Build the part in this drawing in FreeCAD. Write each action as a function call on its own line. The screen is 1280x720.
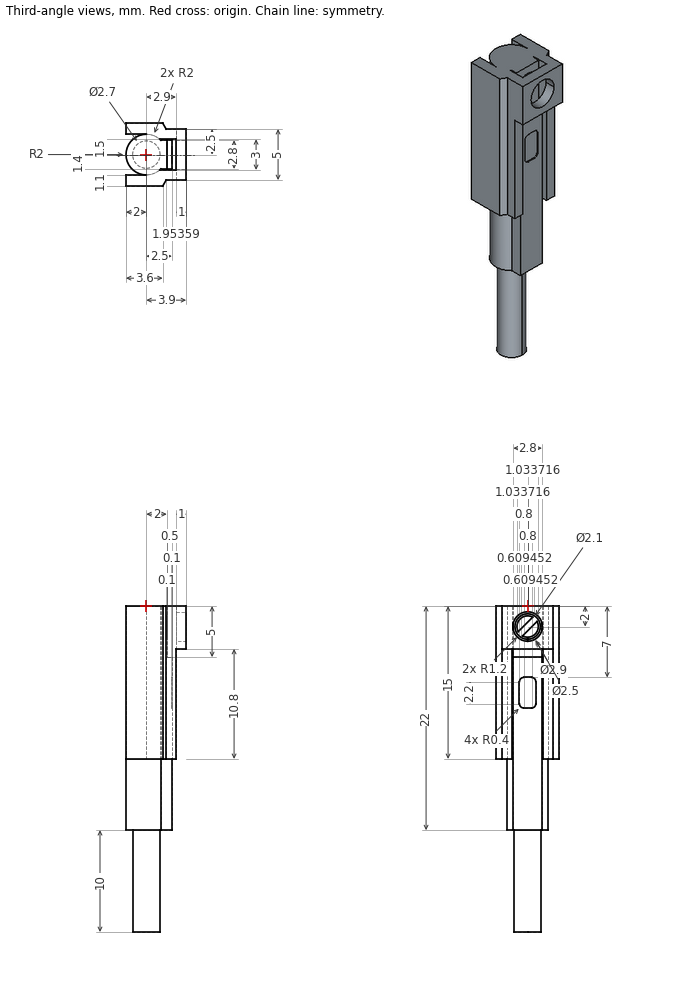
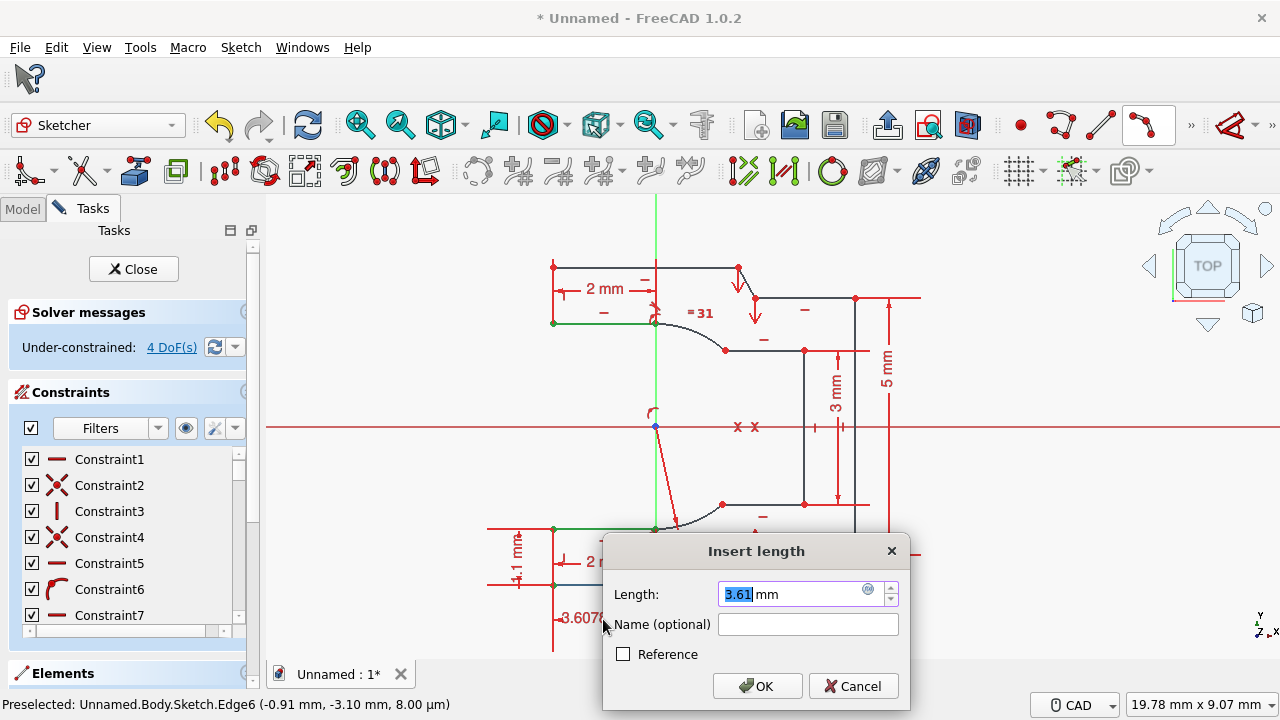
text(3.6)
key(Return)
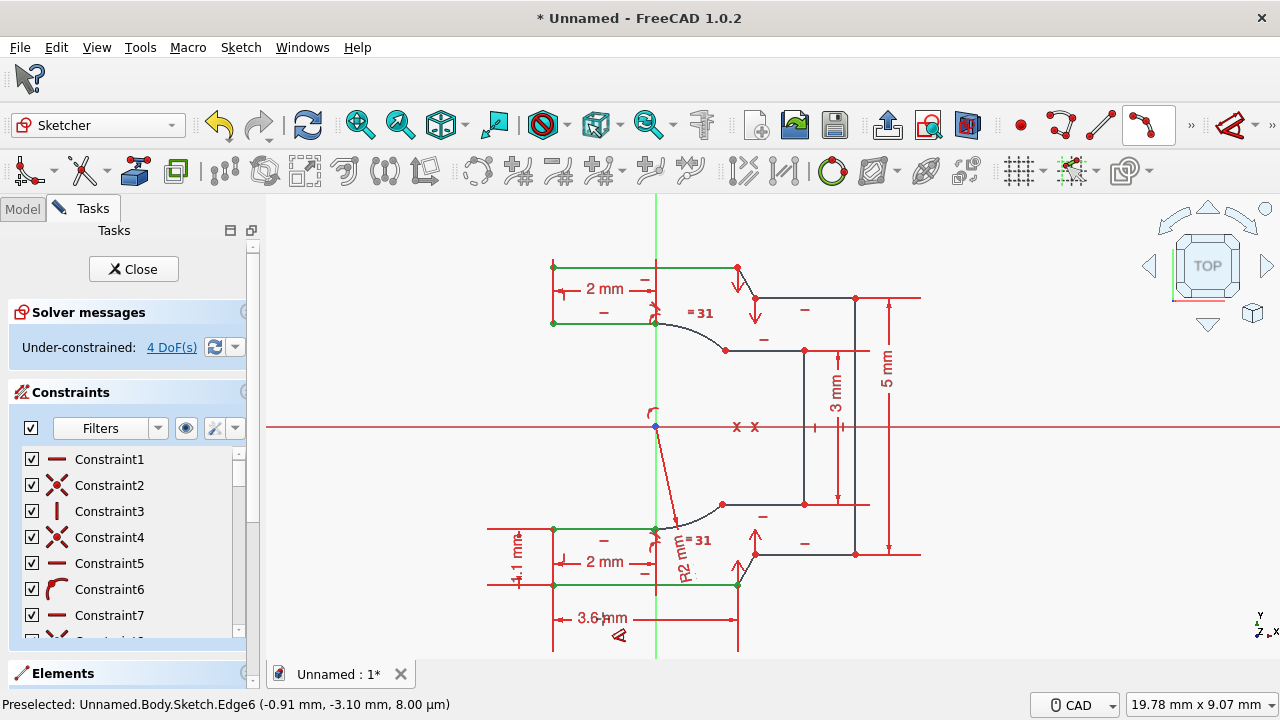
click(725, 351)
click(622, 389)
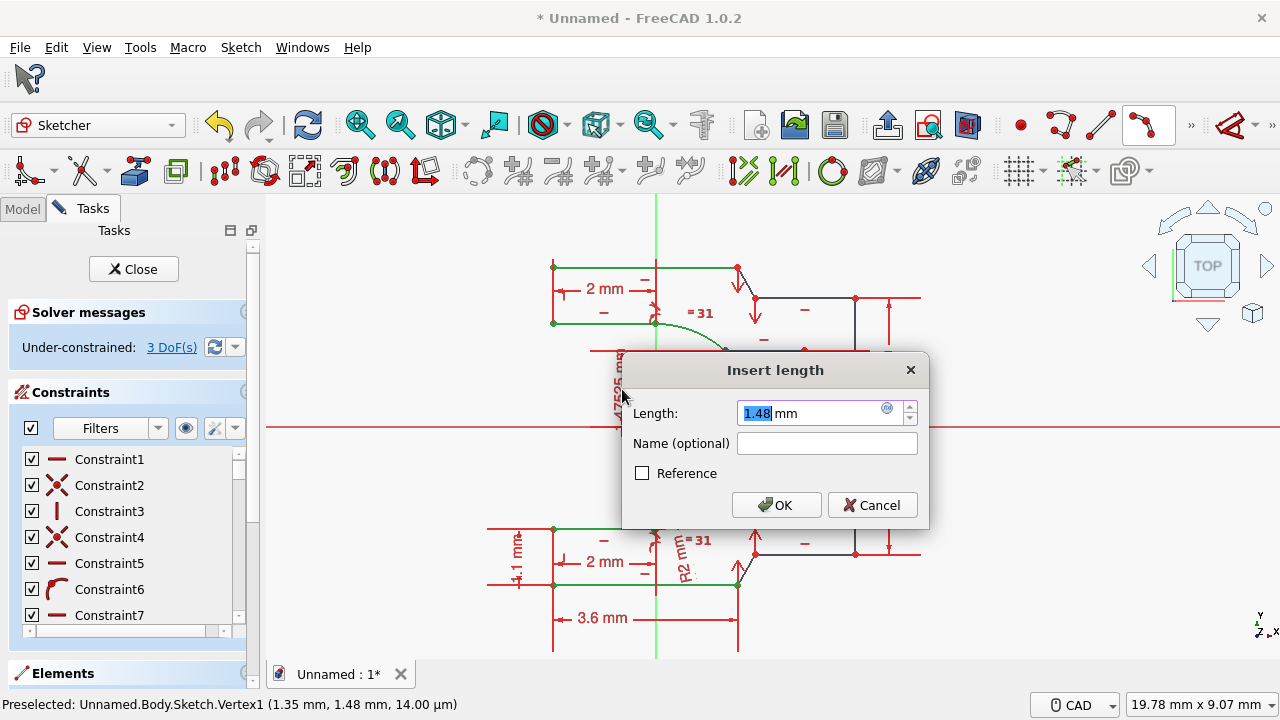
text(1.5)
key(Return)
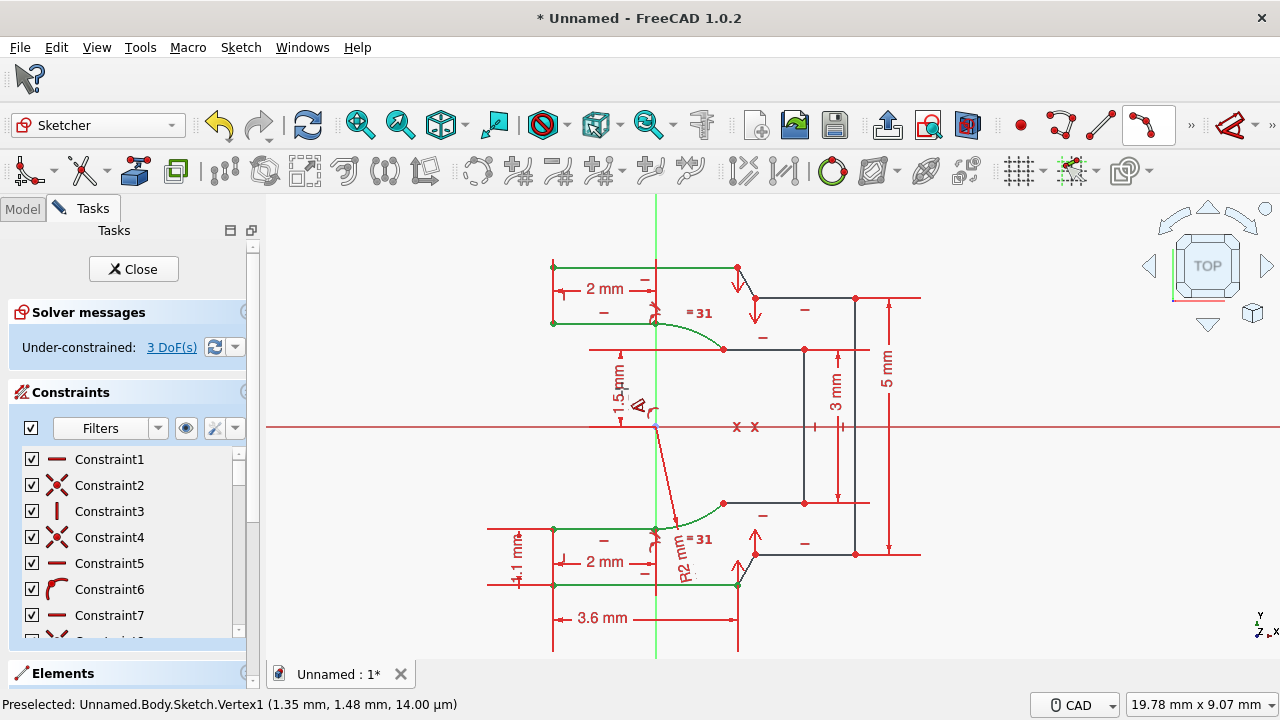
click(804, 350)
click(730, 316)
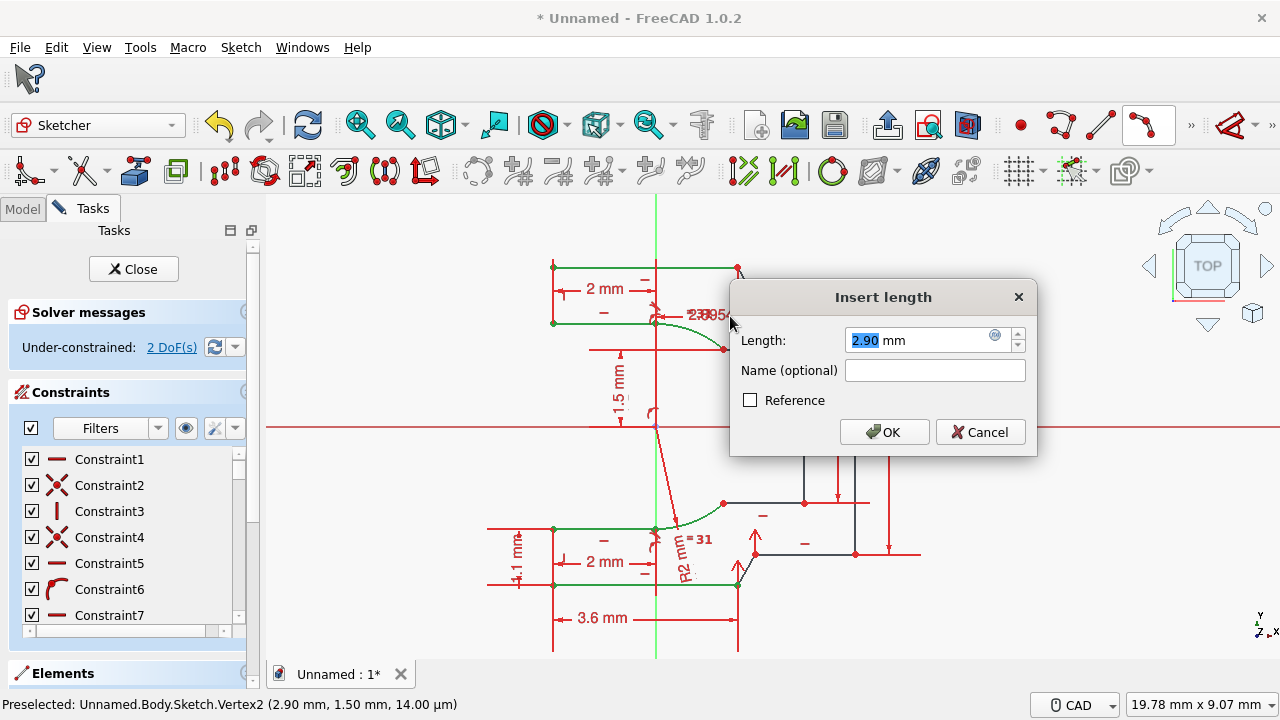
text(2.9)
key(Return)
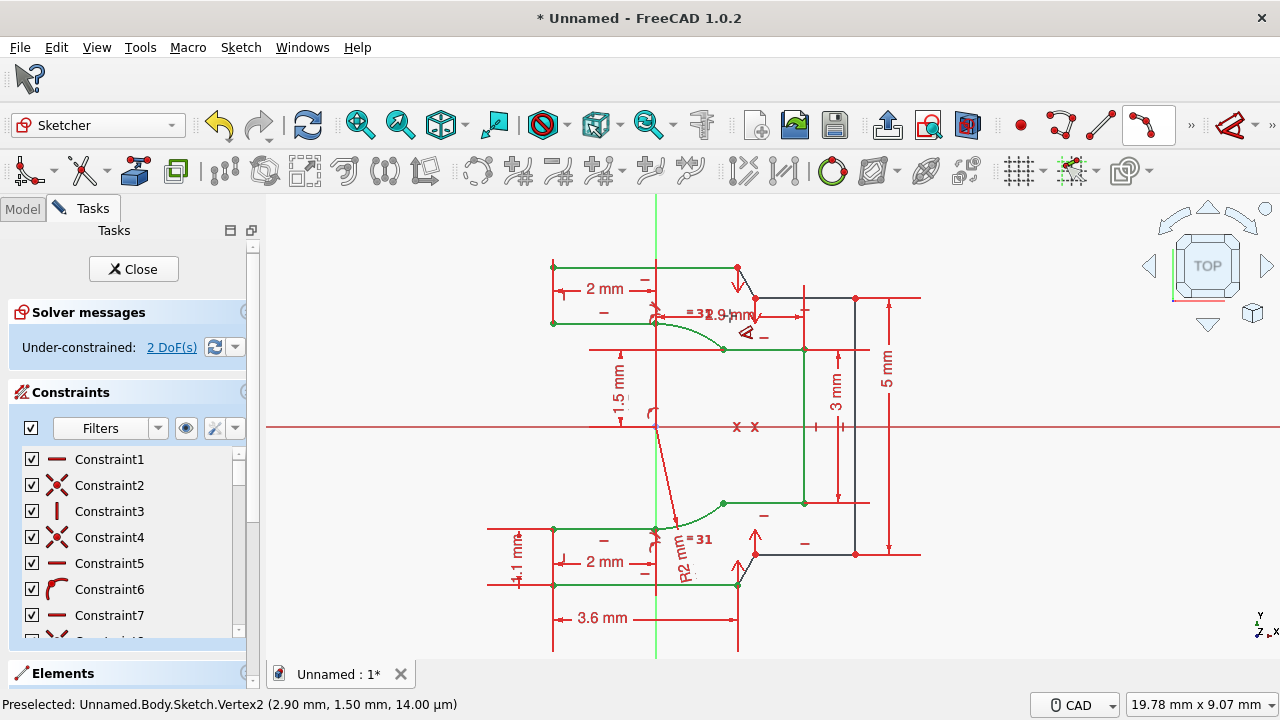
click(855, 555)
click(756, 589)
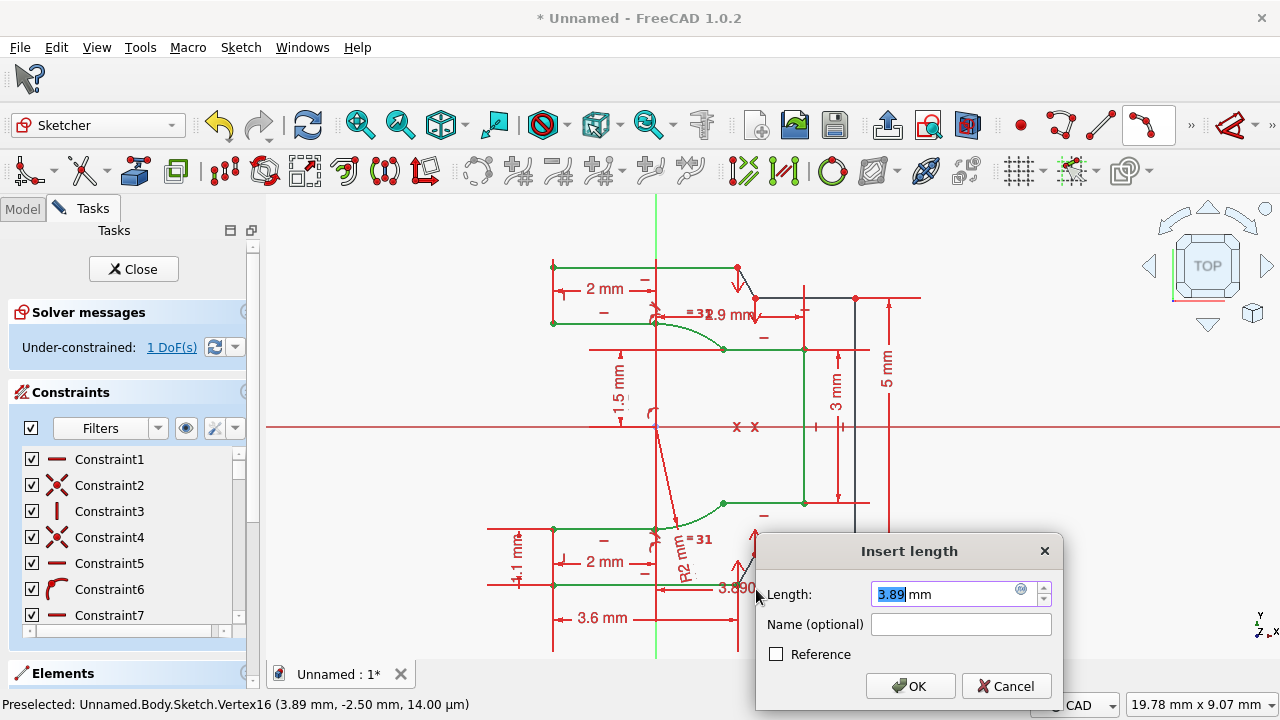
text(3.9)
key(Return)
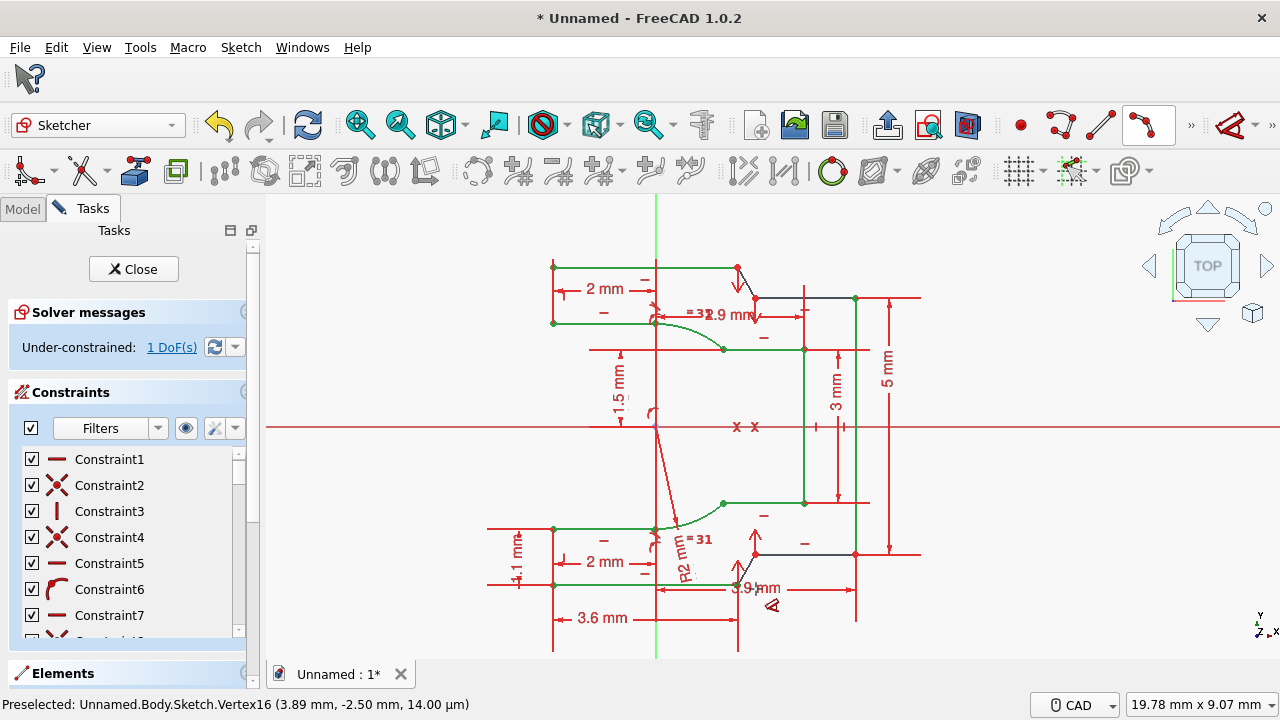
click(785, 555)
click(829, 589)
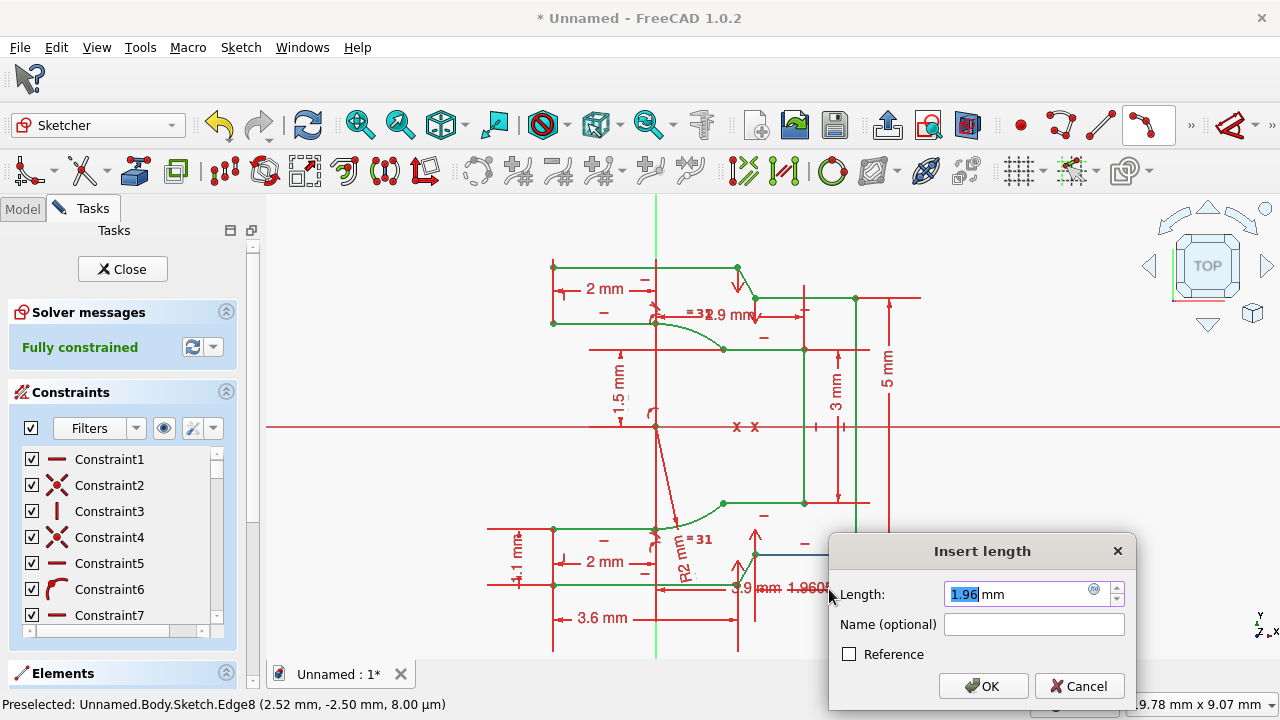
text(1.95359)
key(Return)
key(Escape)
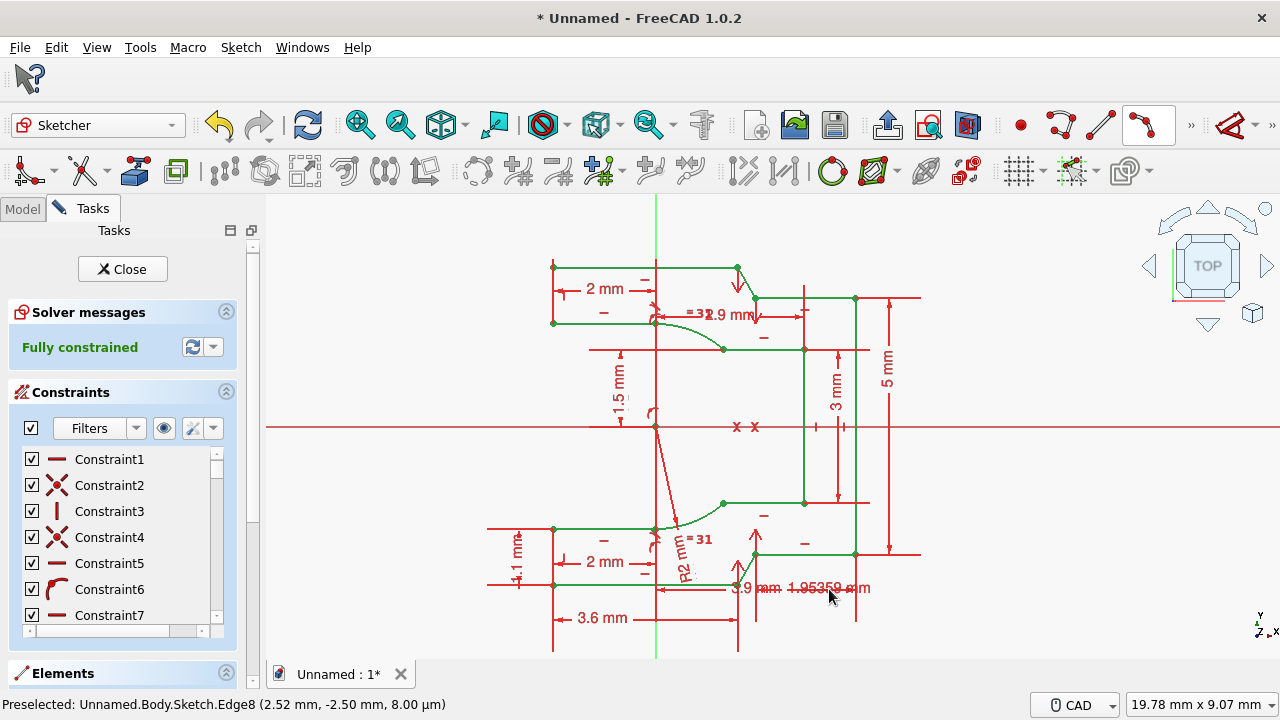
click(123, 269)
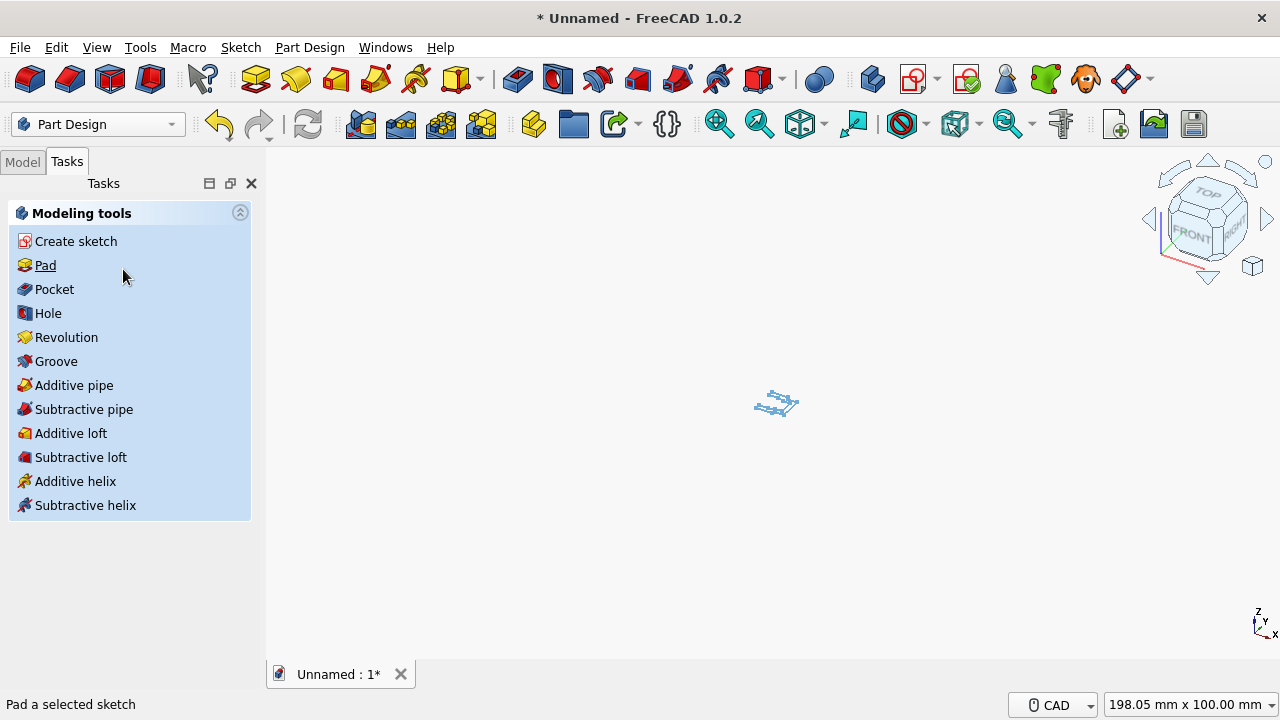
click(256, 80)